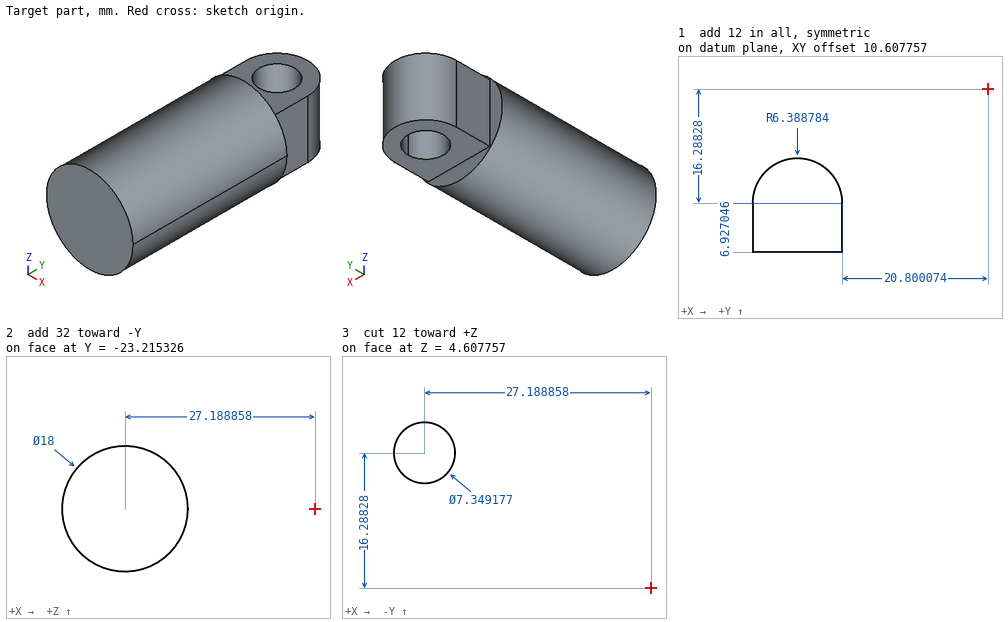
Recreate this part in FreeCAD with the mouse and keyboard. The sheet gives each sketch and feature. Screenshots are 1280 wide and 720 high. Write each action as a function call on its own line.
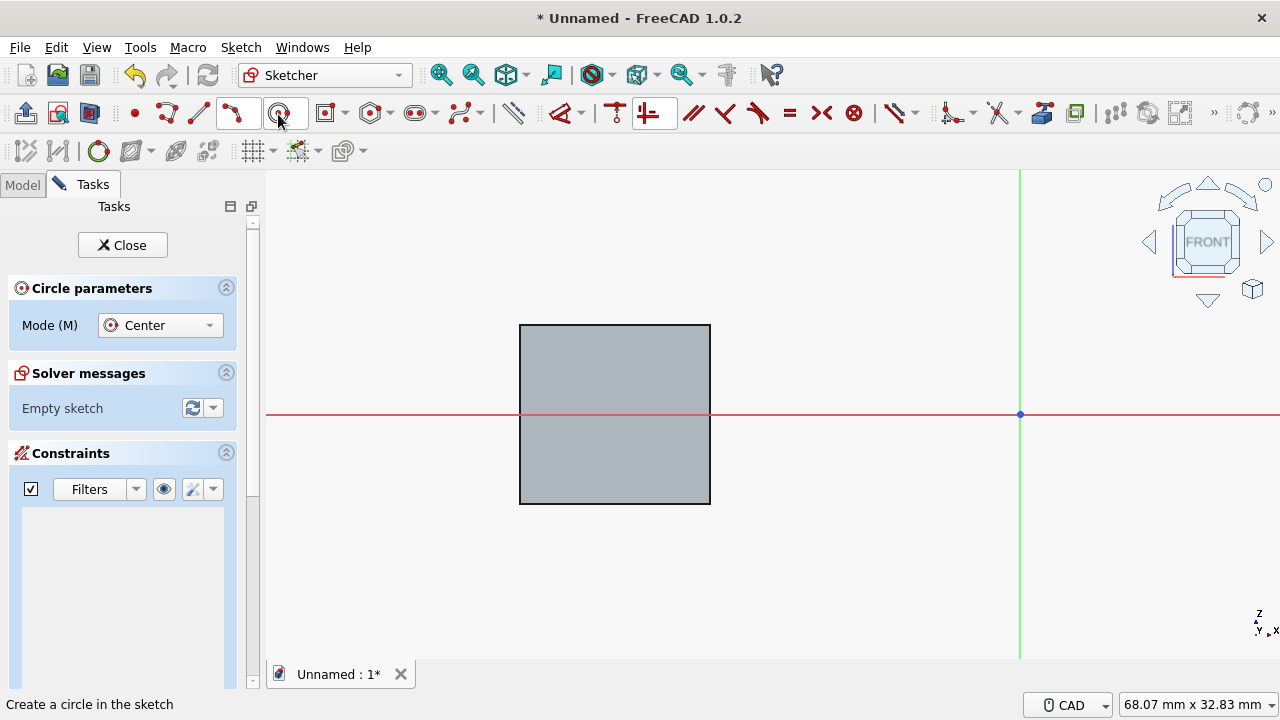
click(615, 415)
move(710, 320)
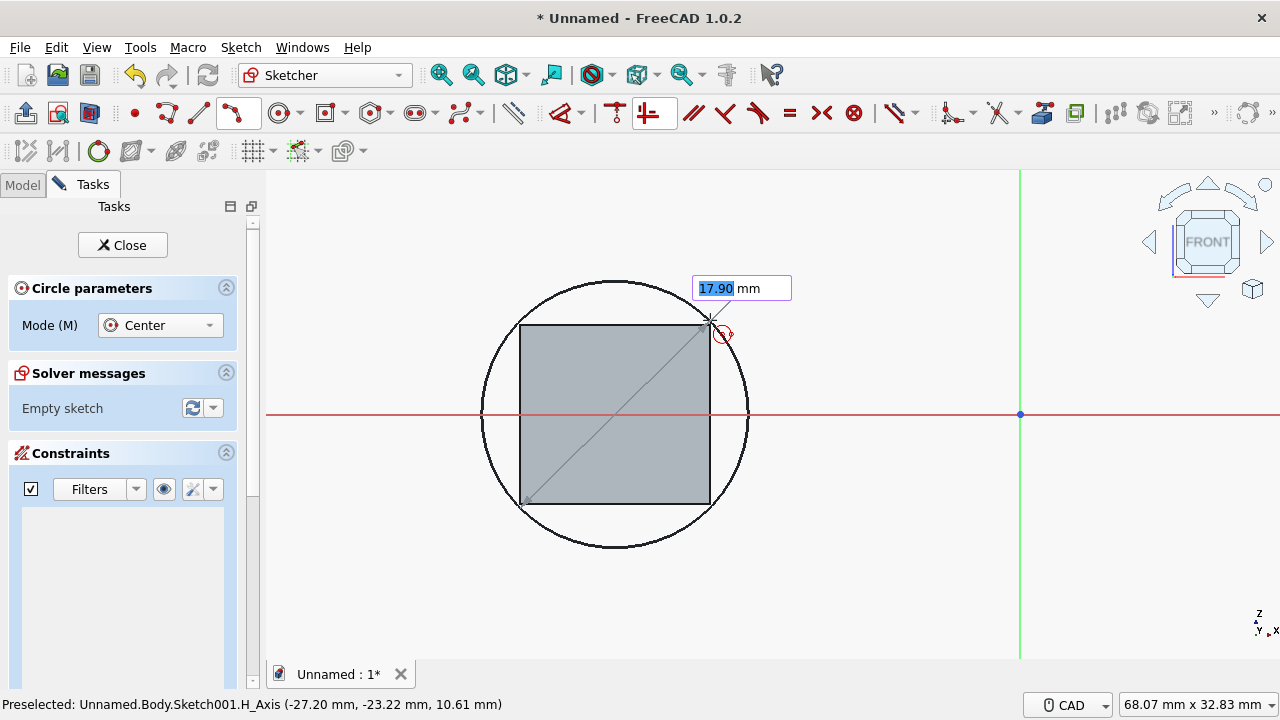
text(18)
key(Return)
key(Escape)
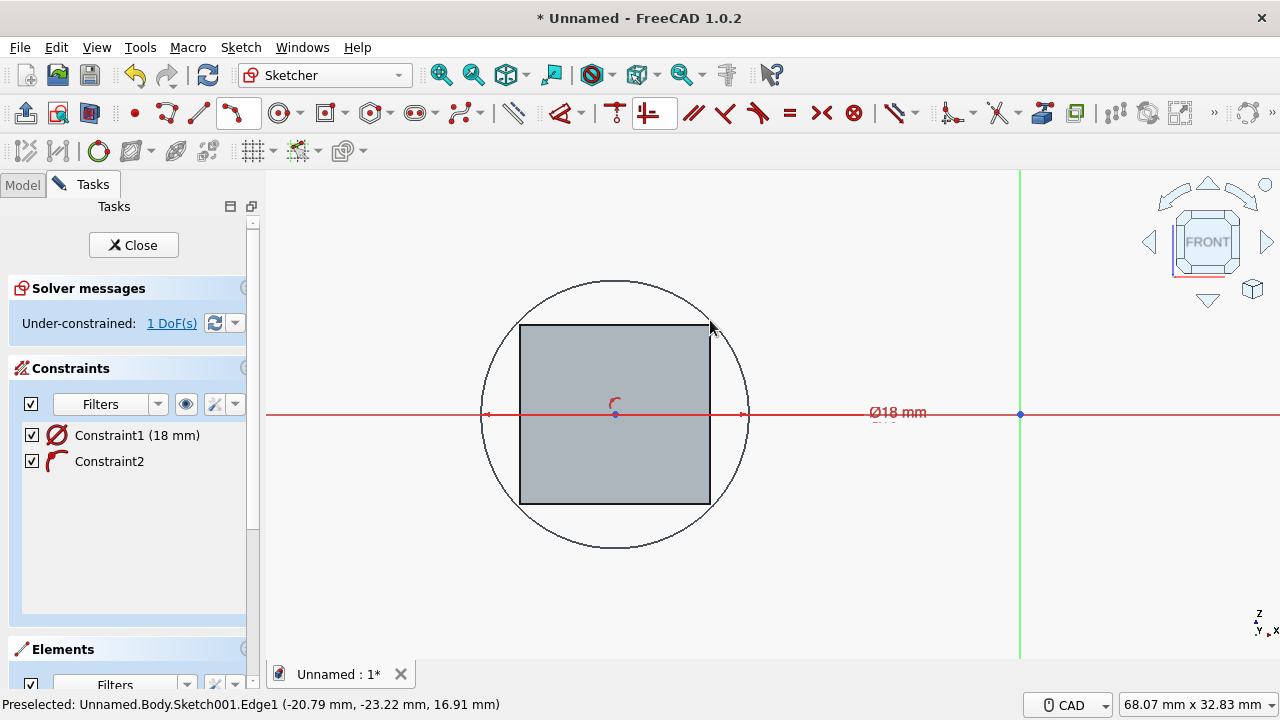
click(560, 114)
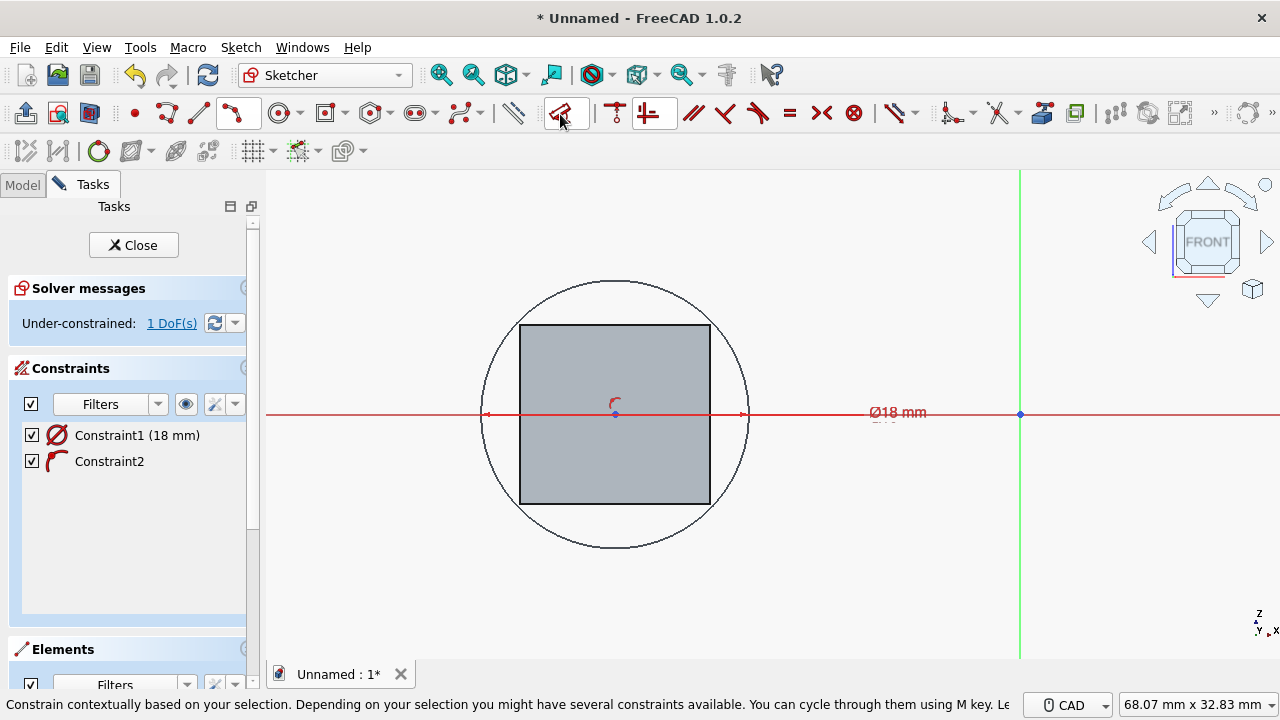
click(615, 415)
click(818, 449)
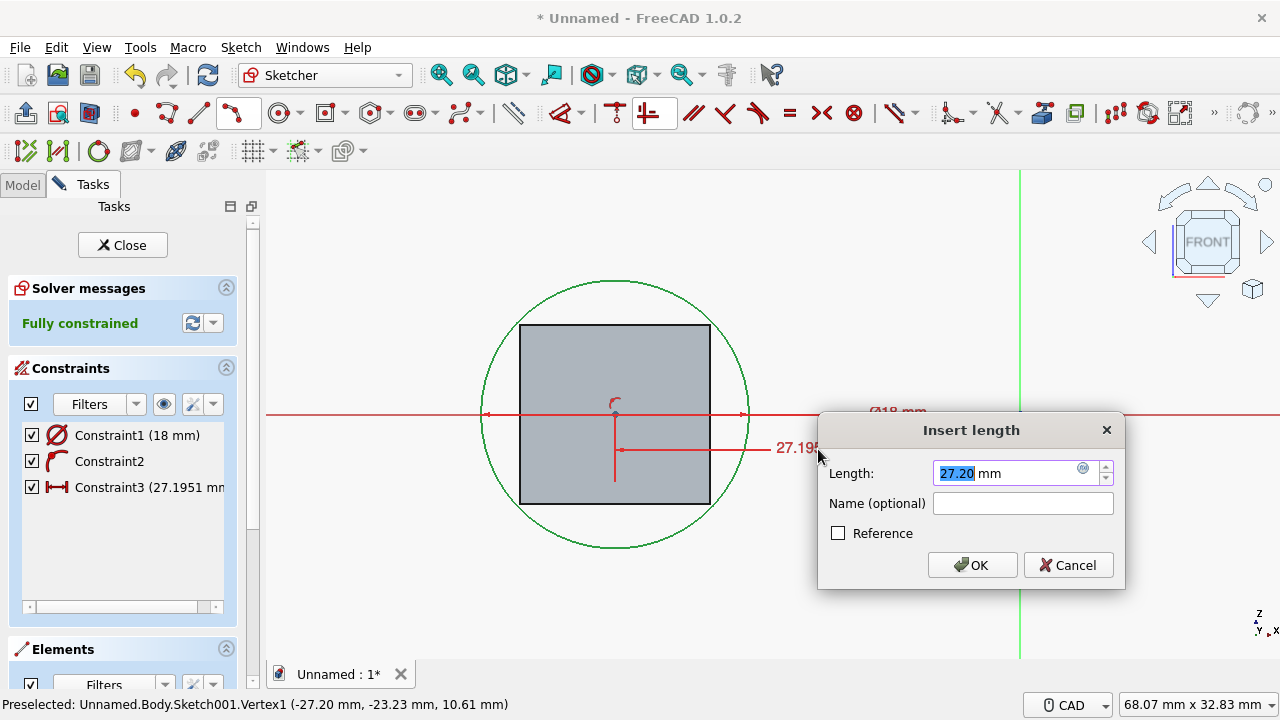
text(27.188858)
key(Return)
key(Escape)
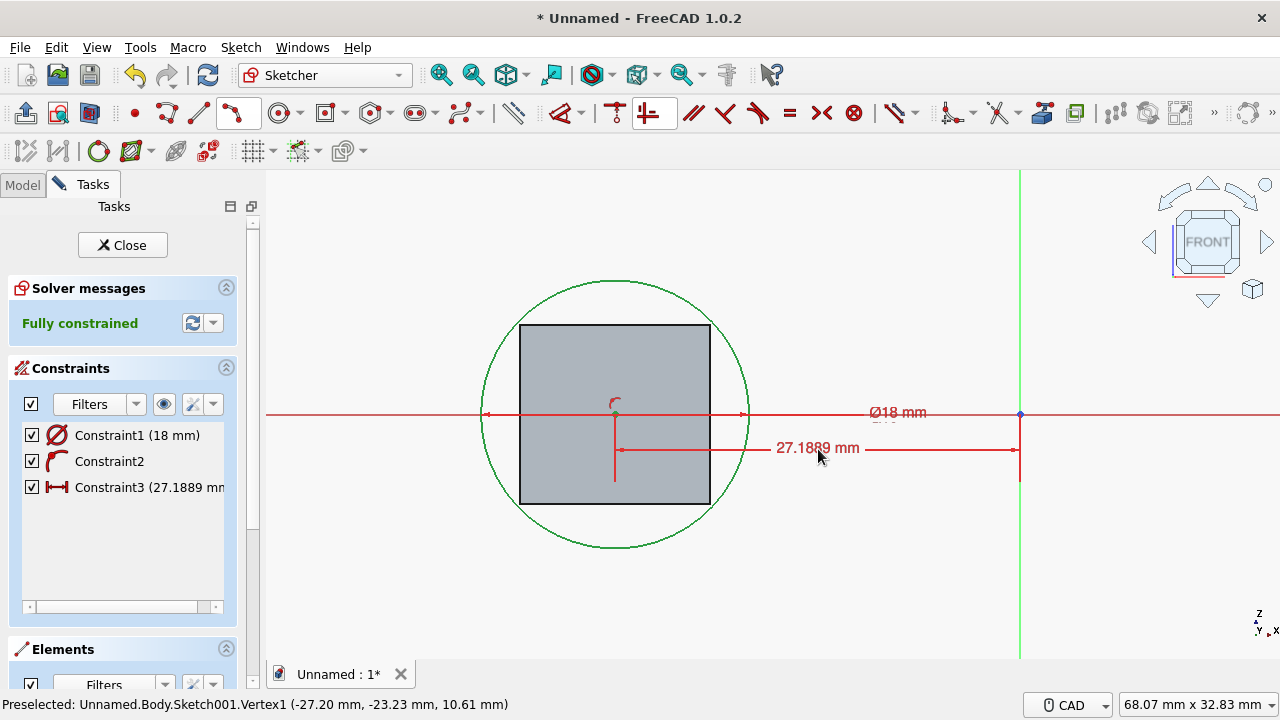
click(123, 245)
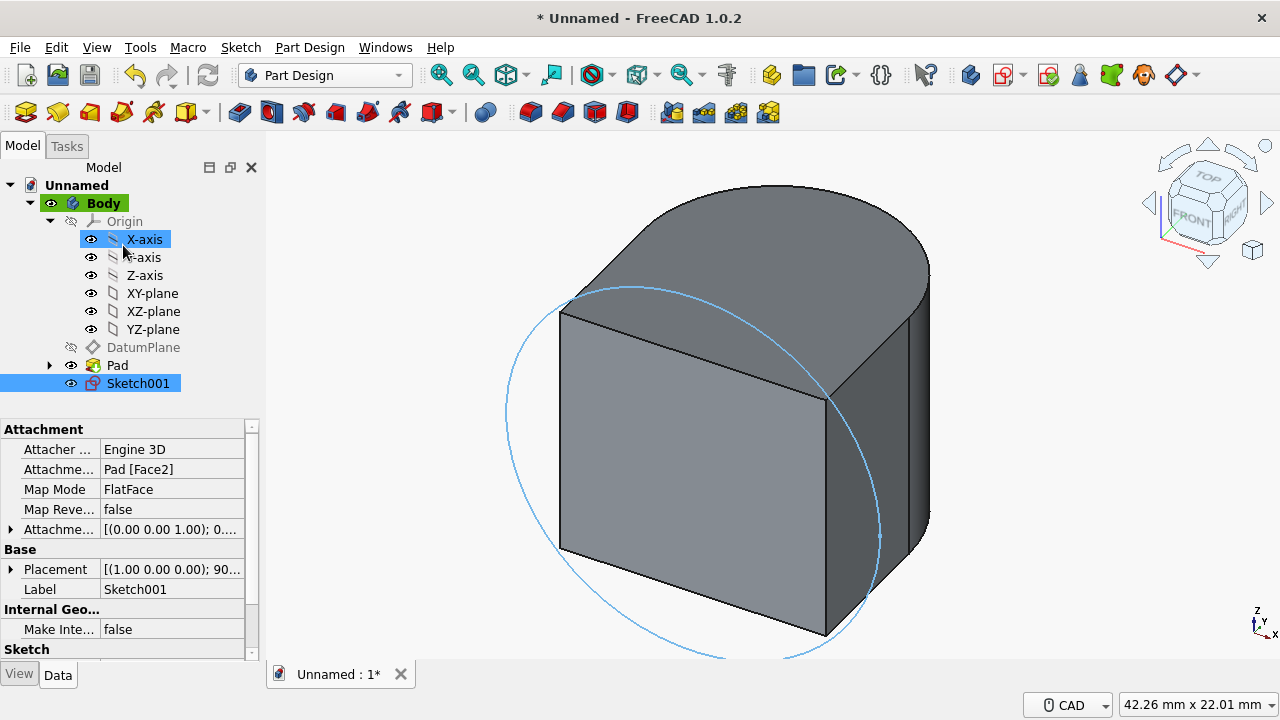
click(26, 112)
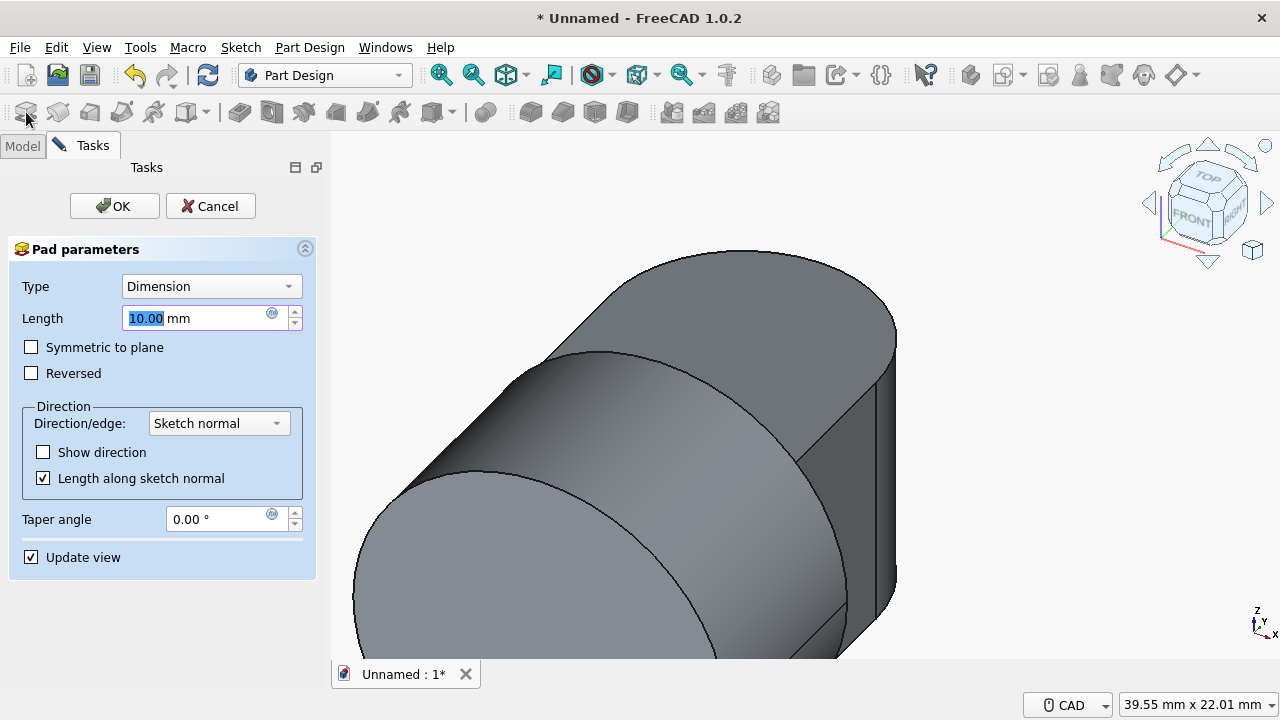
text(32)
key(Tab)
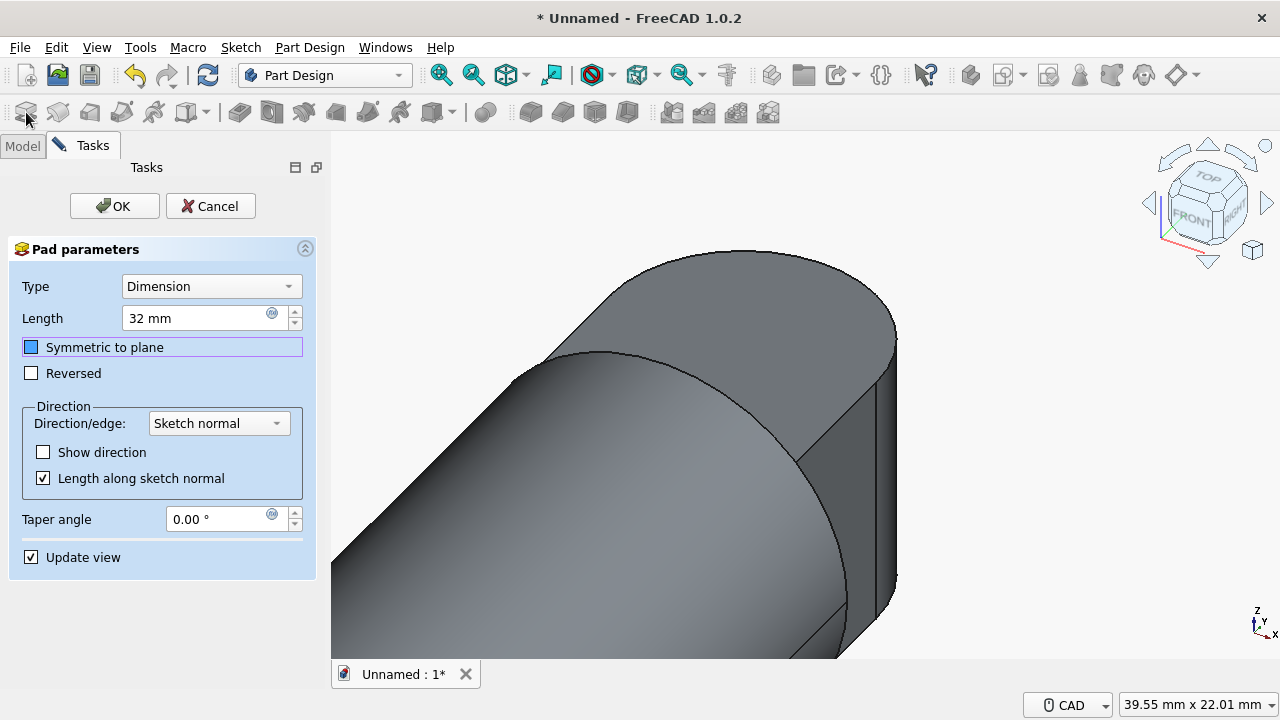
click(115, 206)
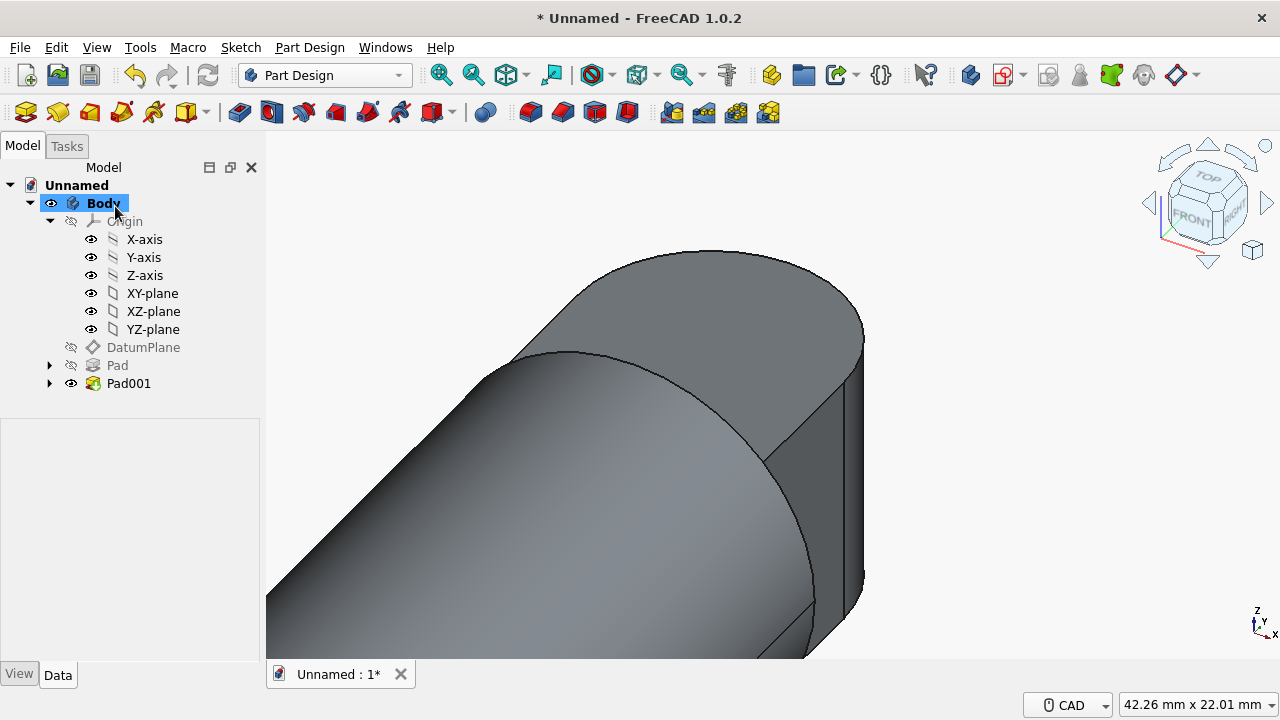
click(442, 76)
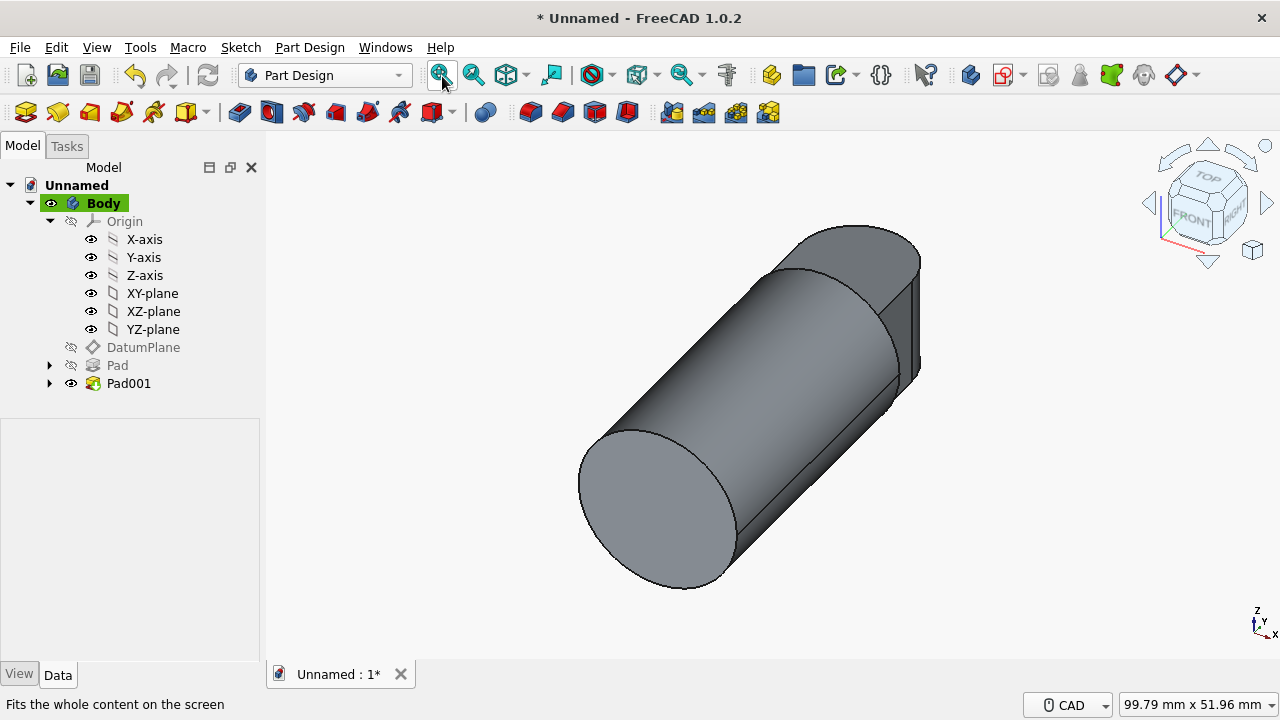
key(5)